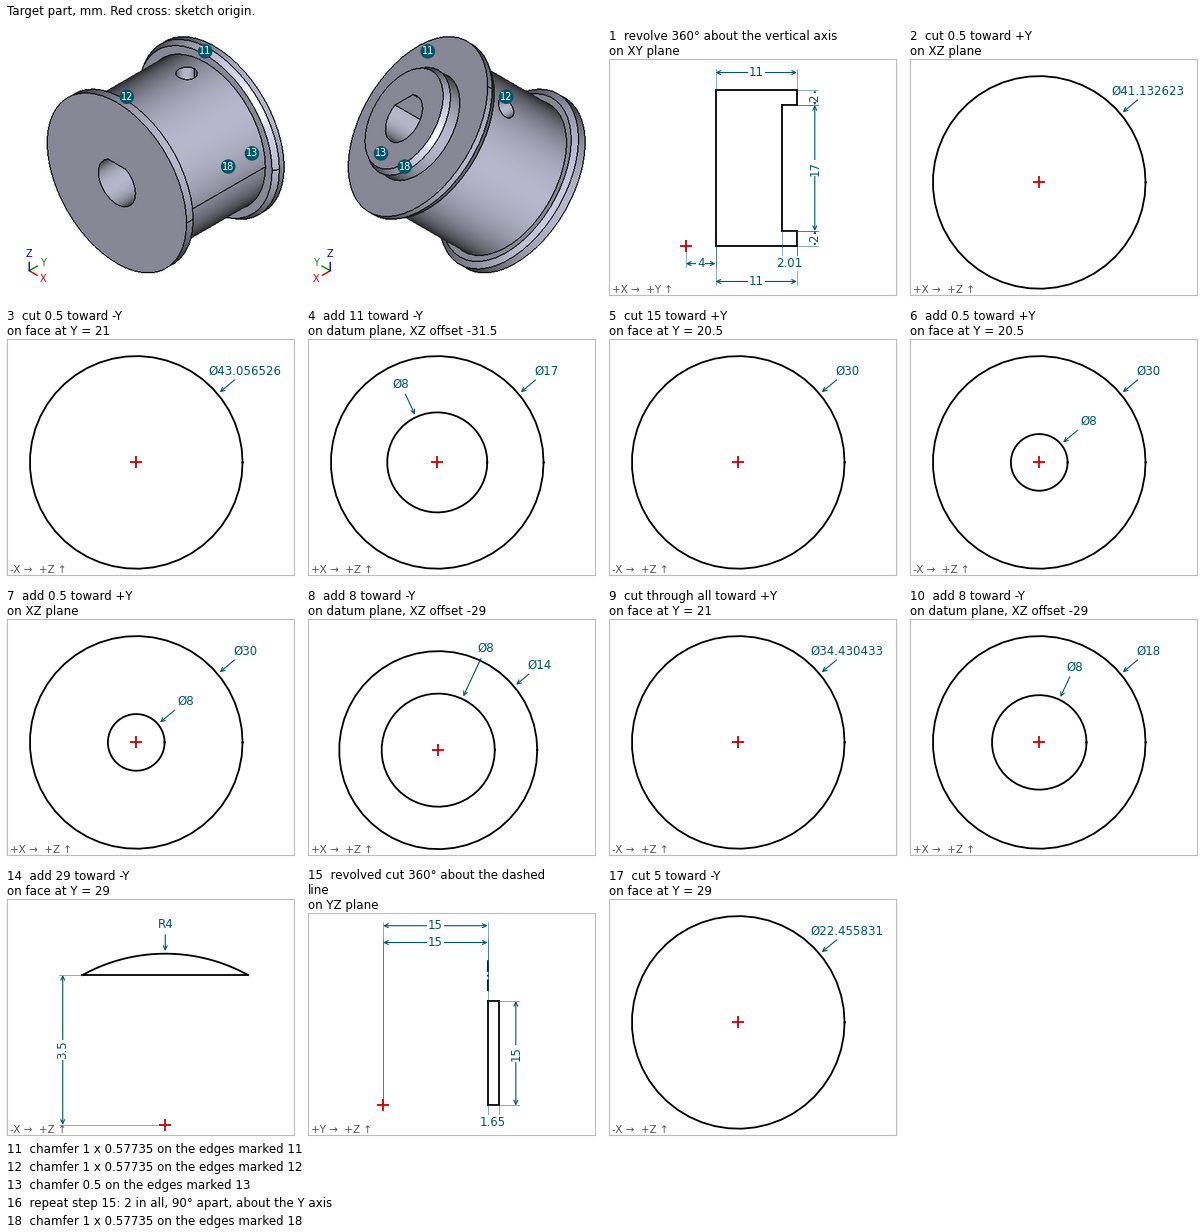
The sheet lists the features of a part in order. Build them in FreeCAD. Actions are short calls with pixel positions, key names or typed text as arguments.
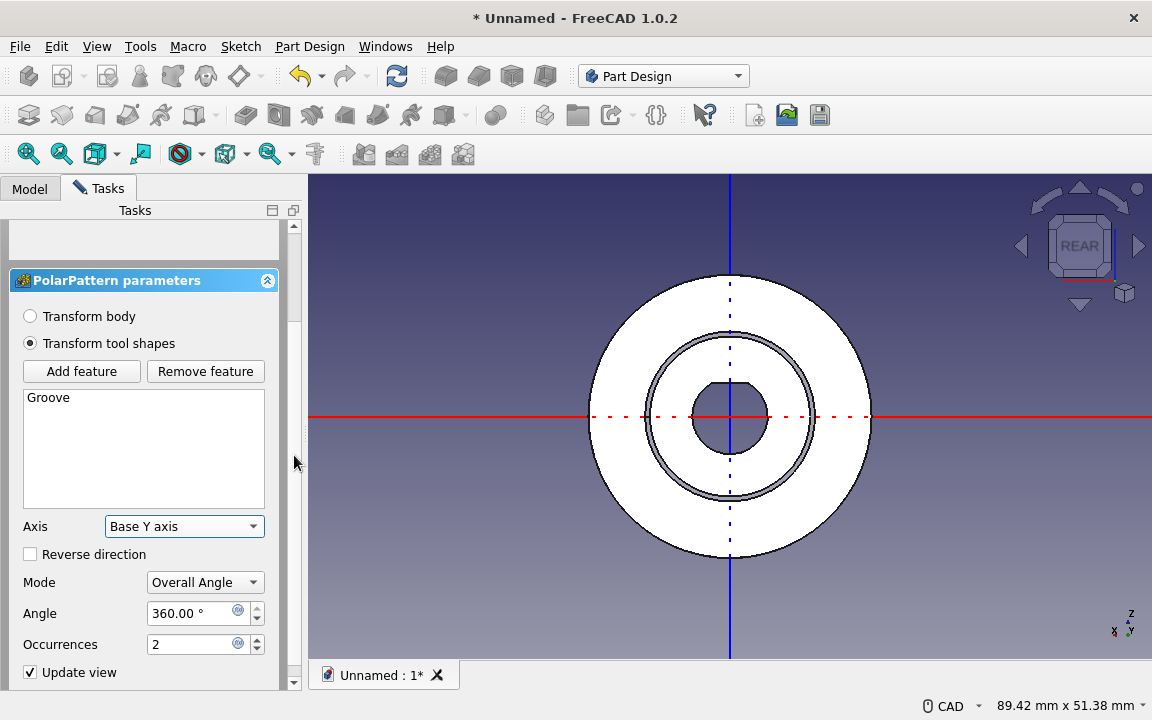
click(206, 582)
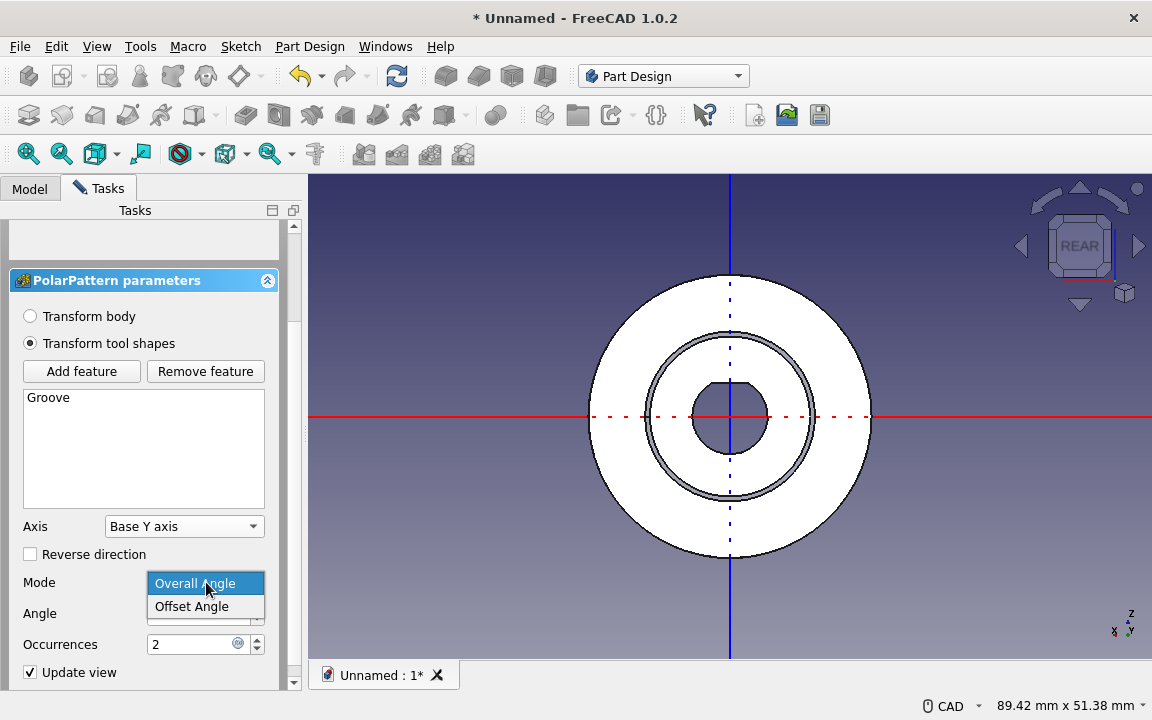
click(204, 606)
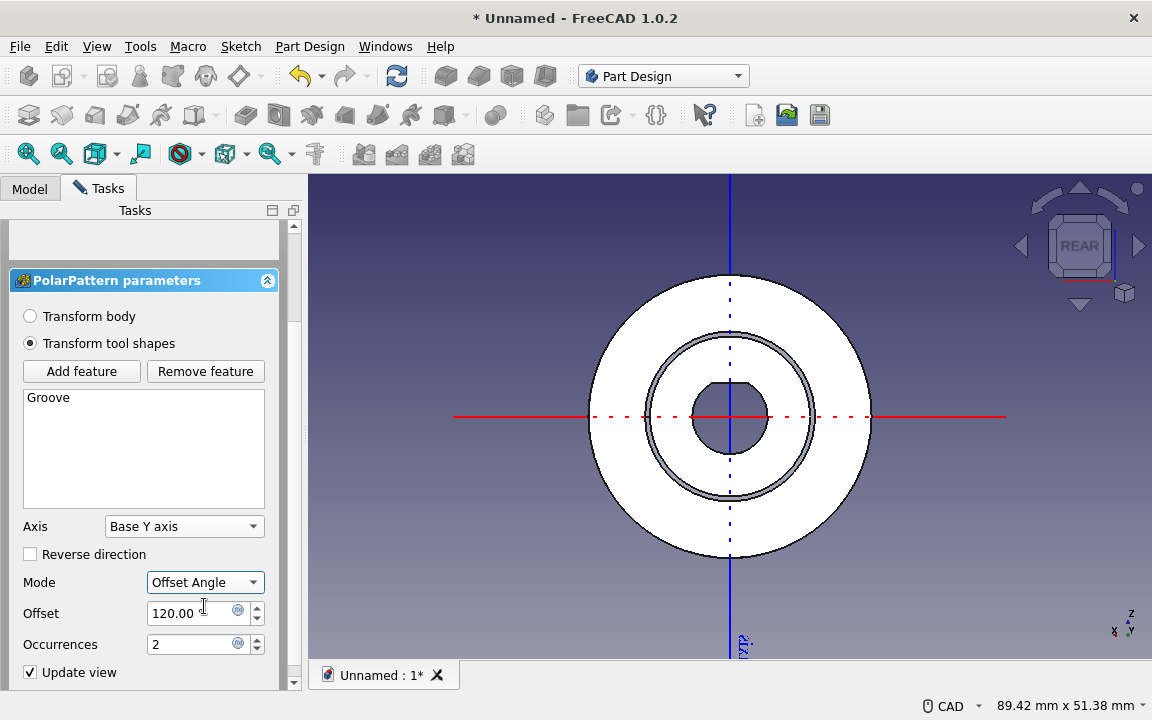
triple_click(199, 614)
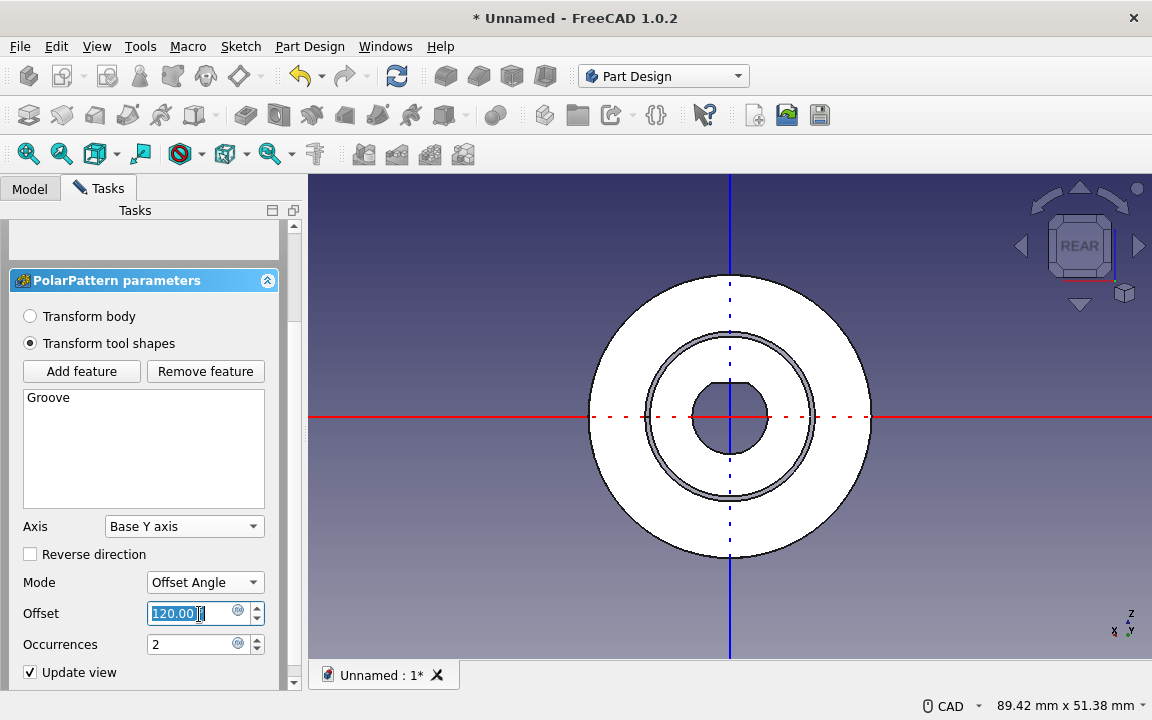
text(90)
key(Tab)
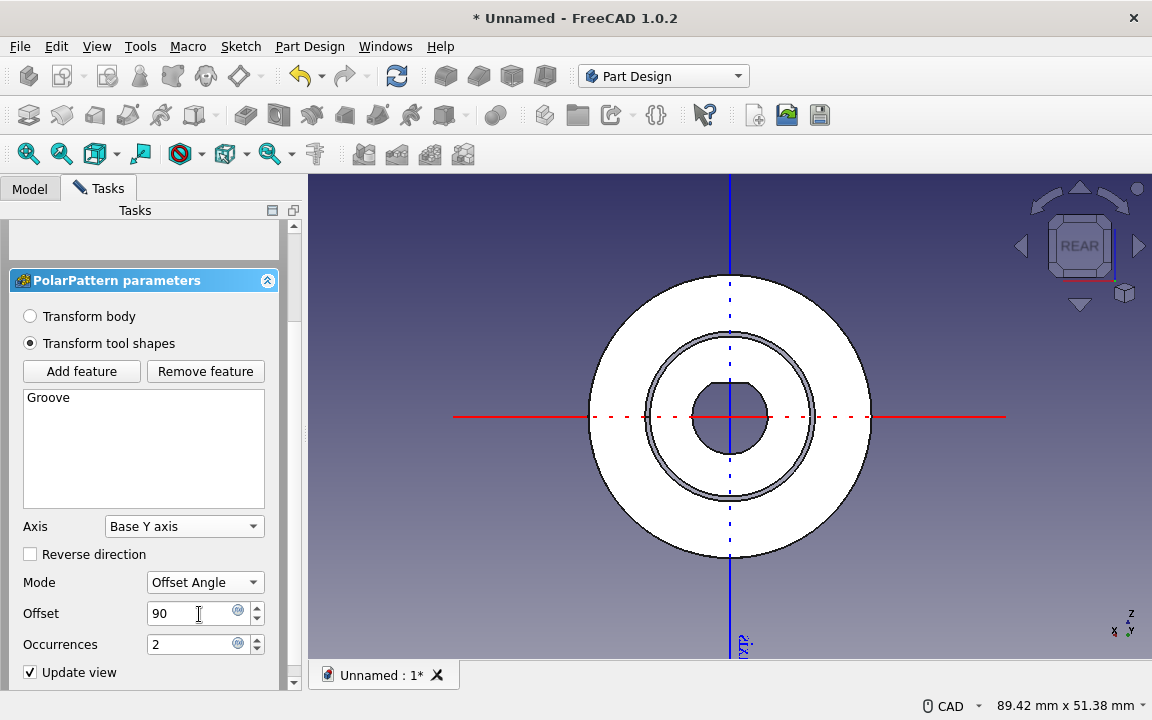
triple_click(199, 644)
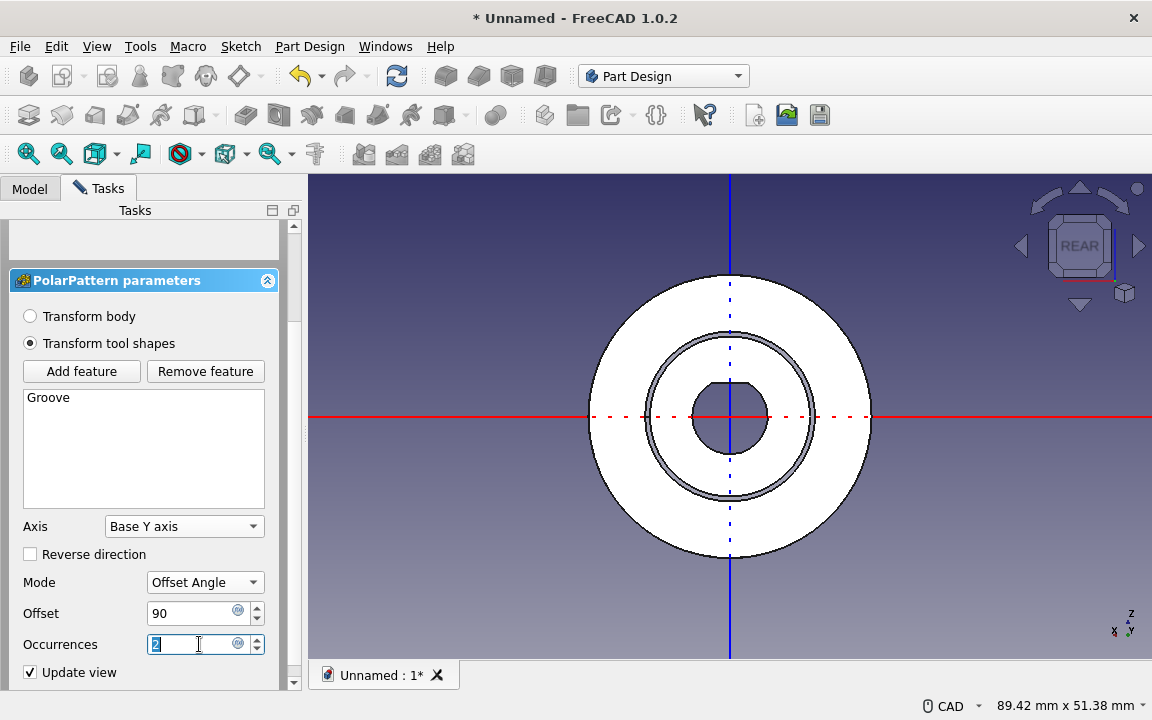
text(2)
key(Tab)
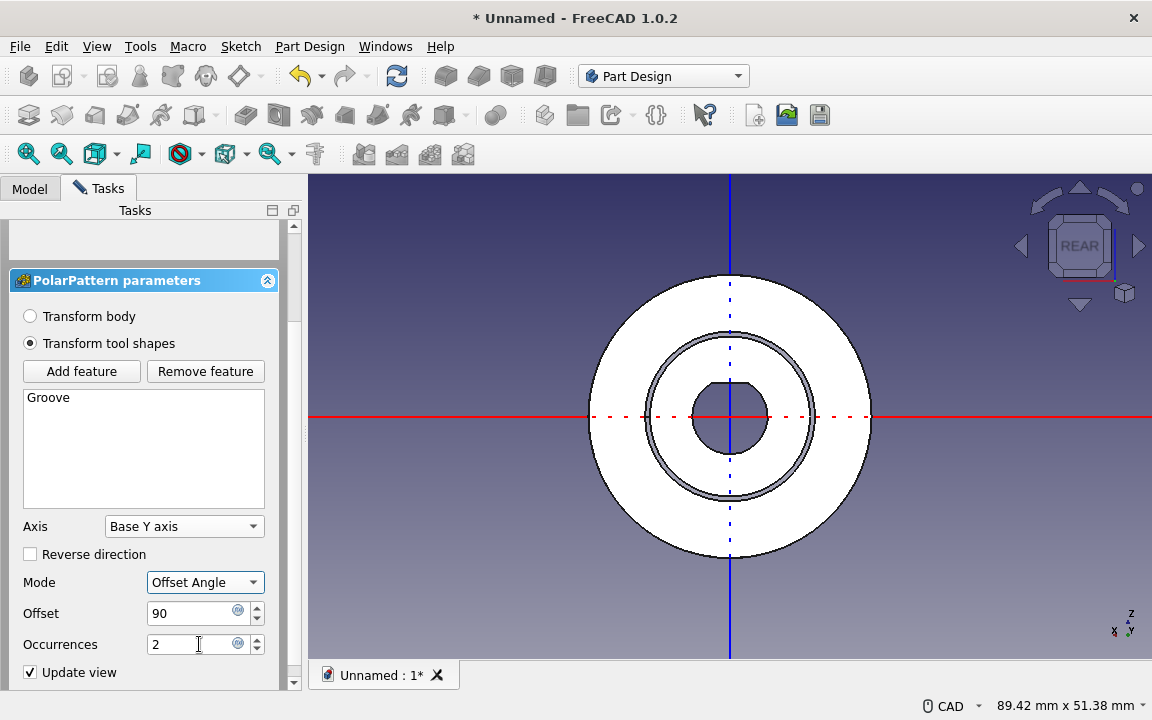
click(31, 554)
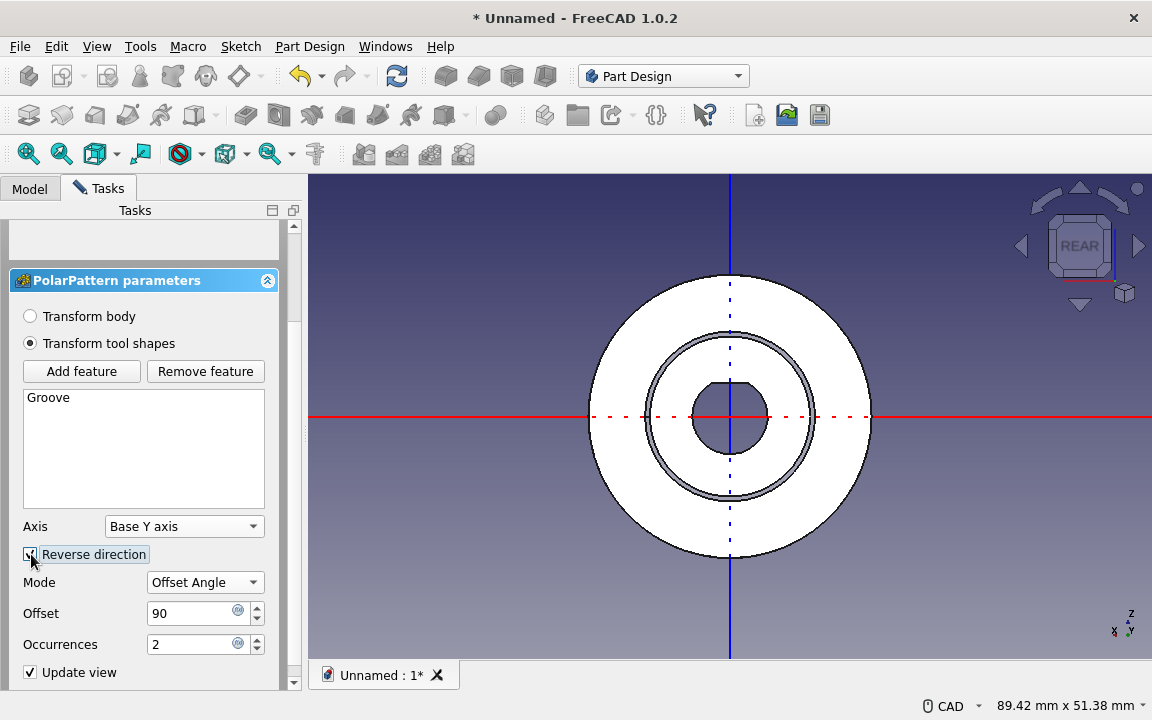
scroll(294, 455, up, 3)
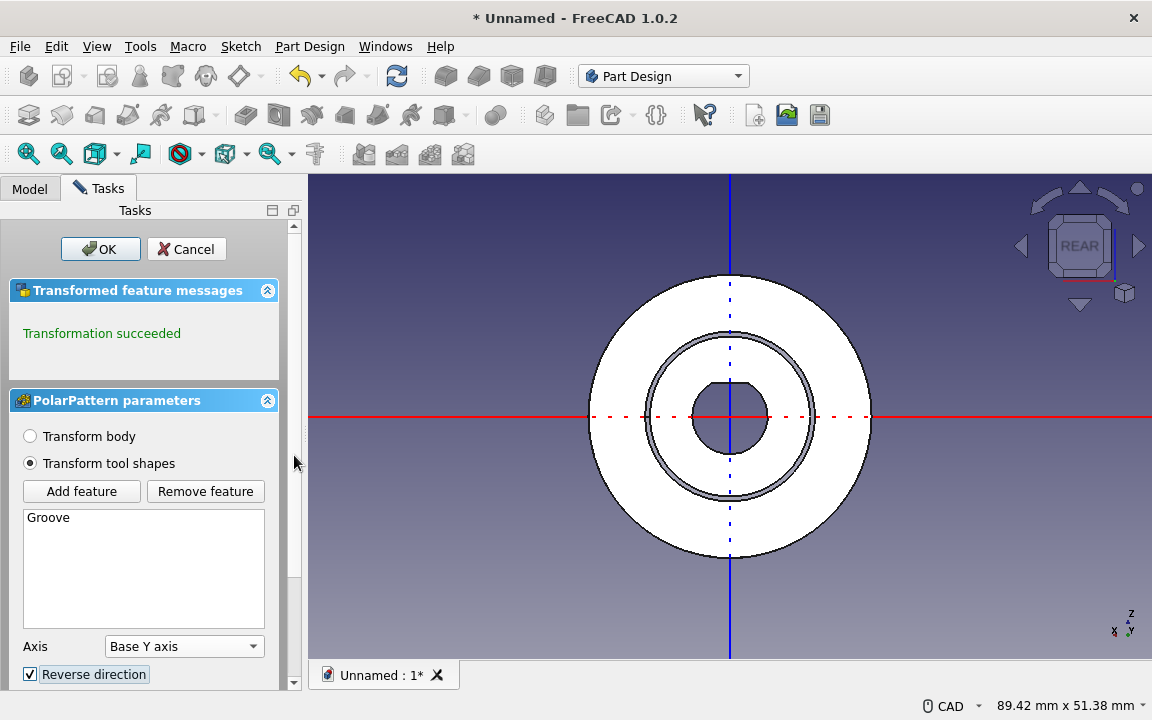
click(101, 249)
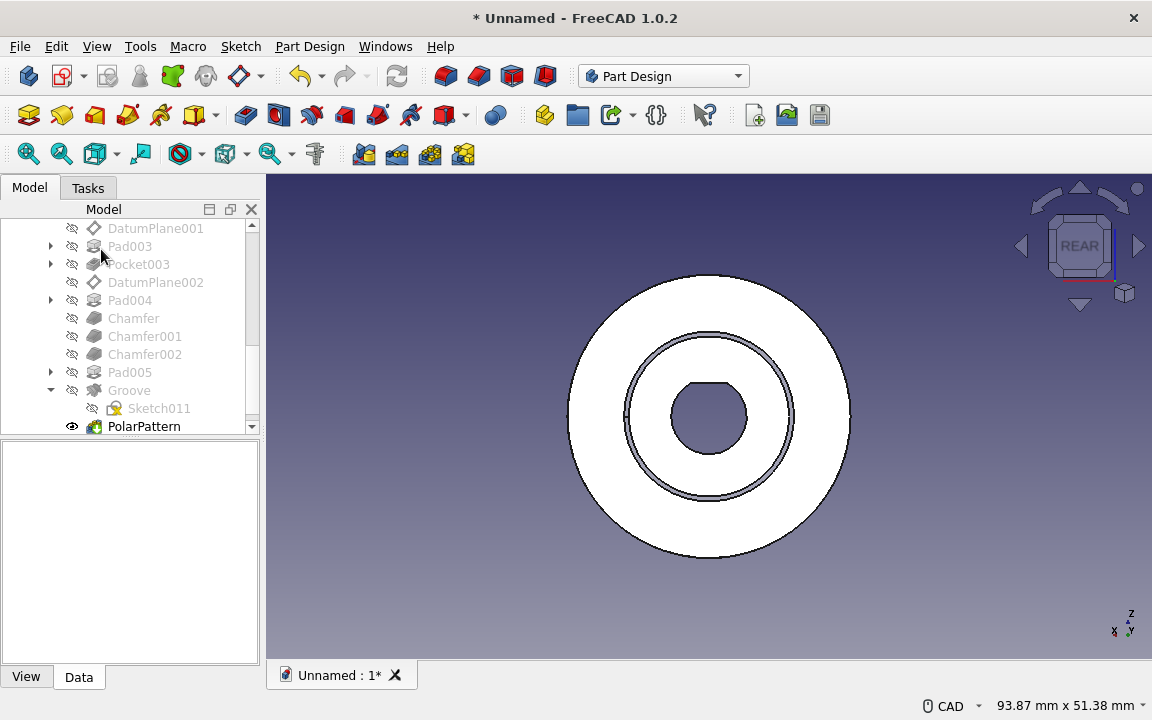
click(755, 461)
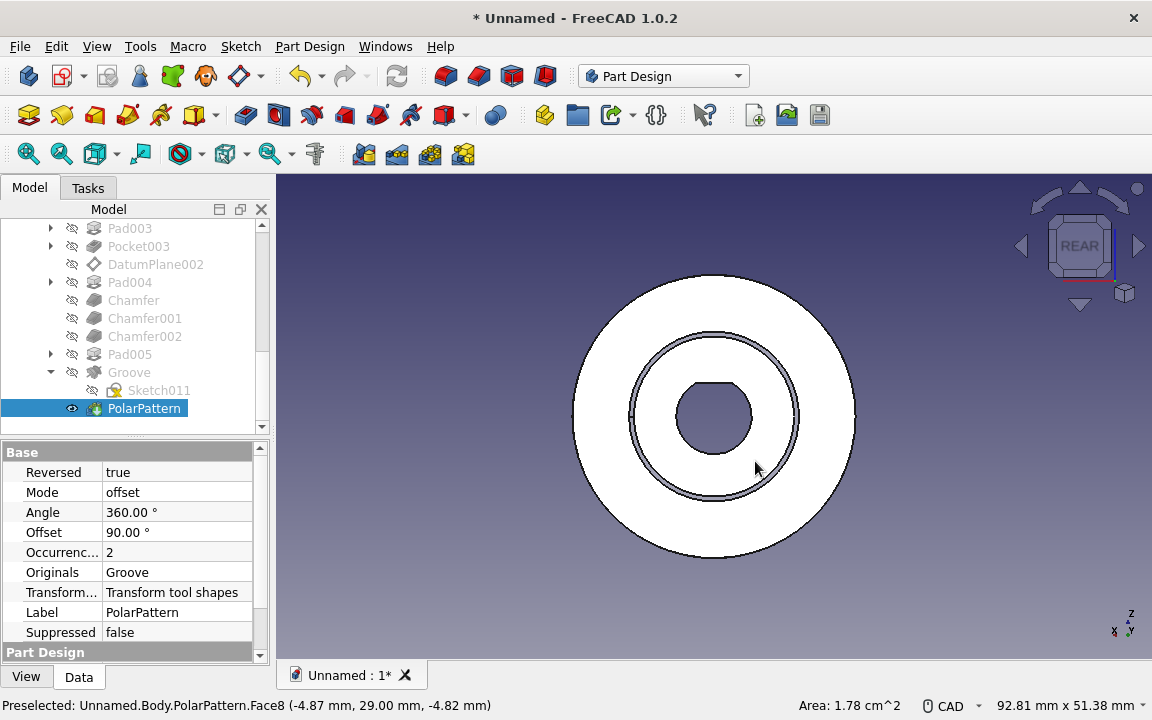
click(62, 76)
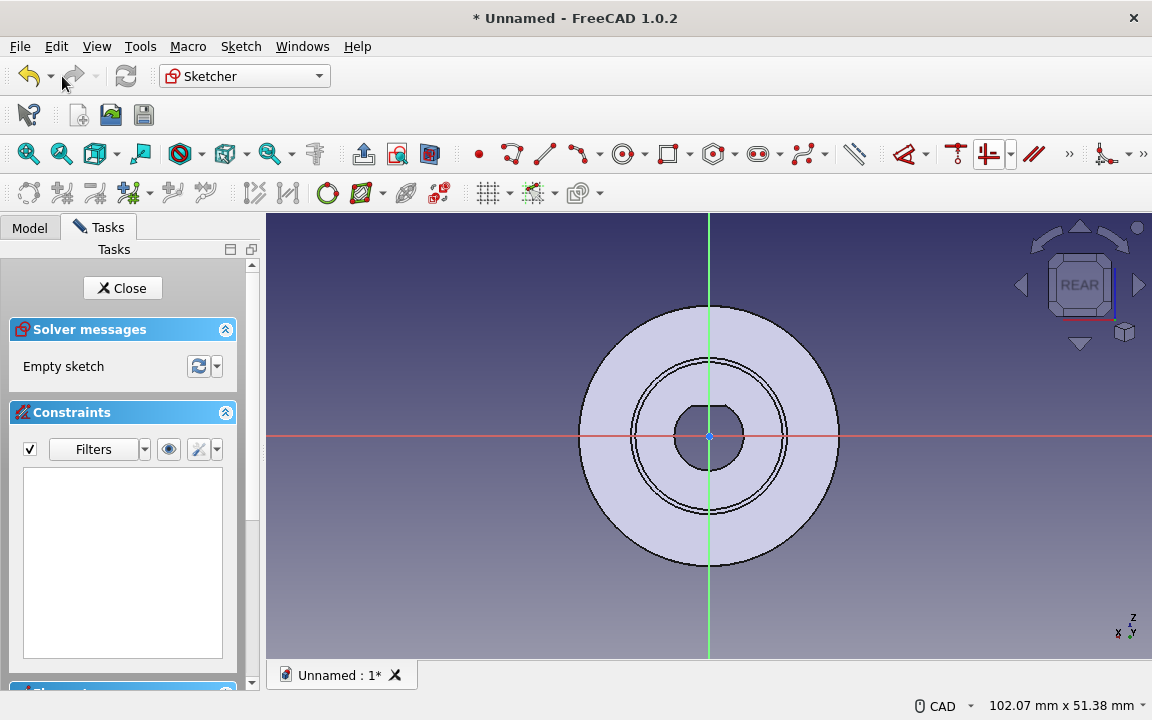
scroll(848, 436, up, 2)